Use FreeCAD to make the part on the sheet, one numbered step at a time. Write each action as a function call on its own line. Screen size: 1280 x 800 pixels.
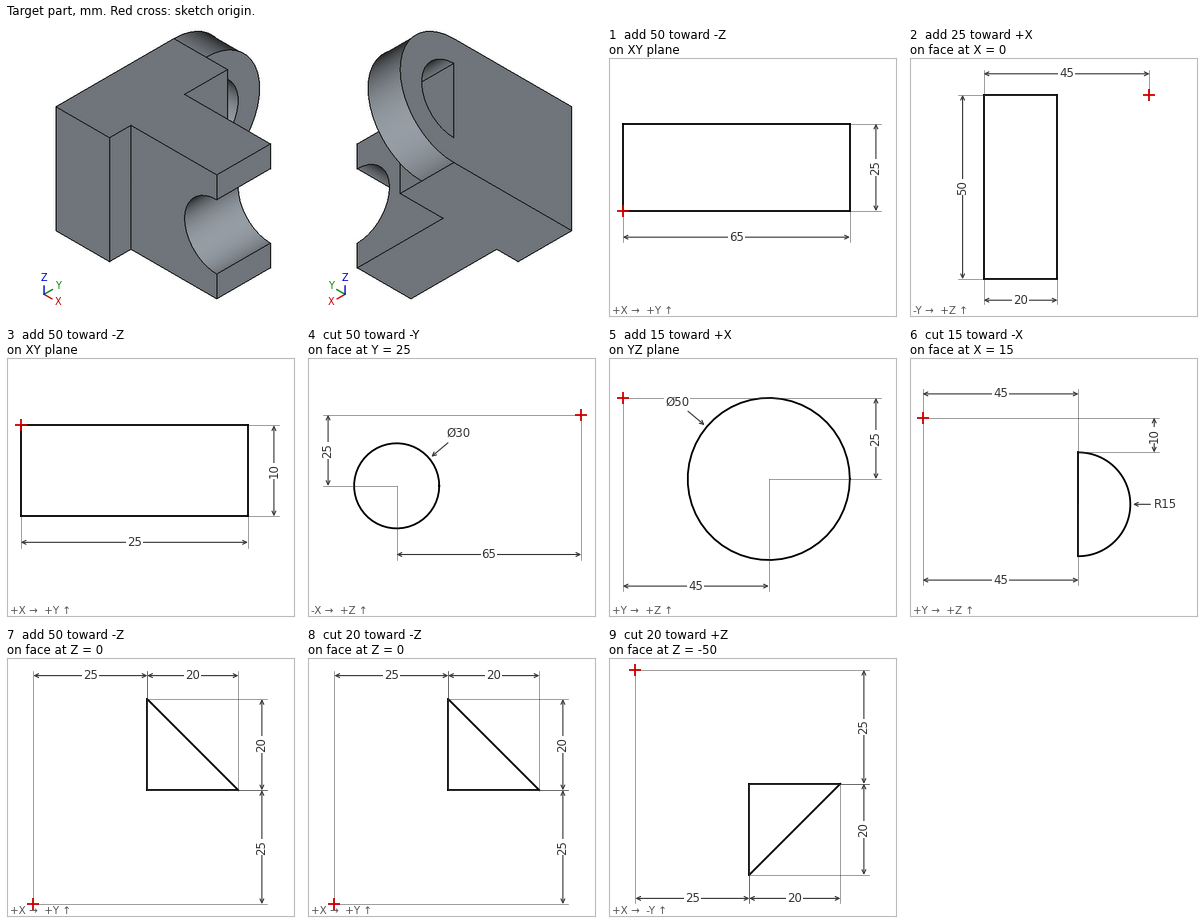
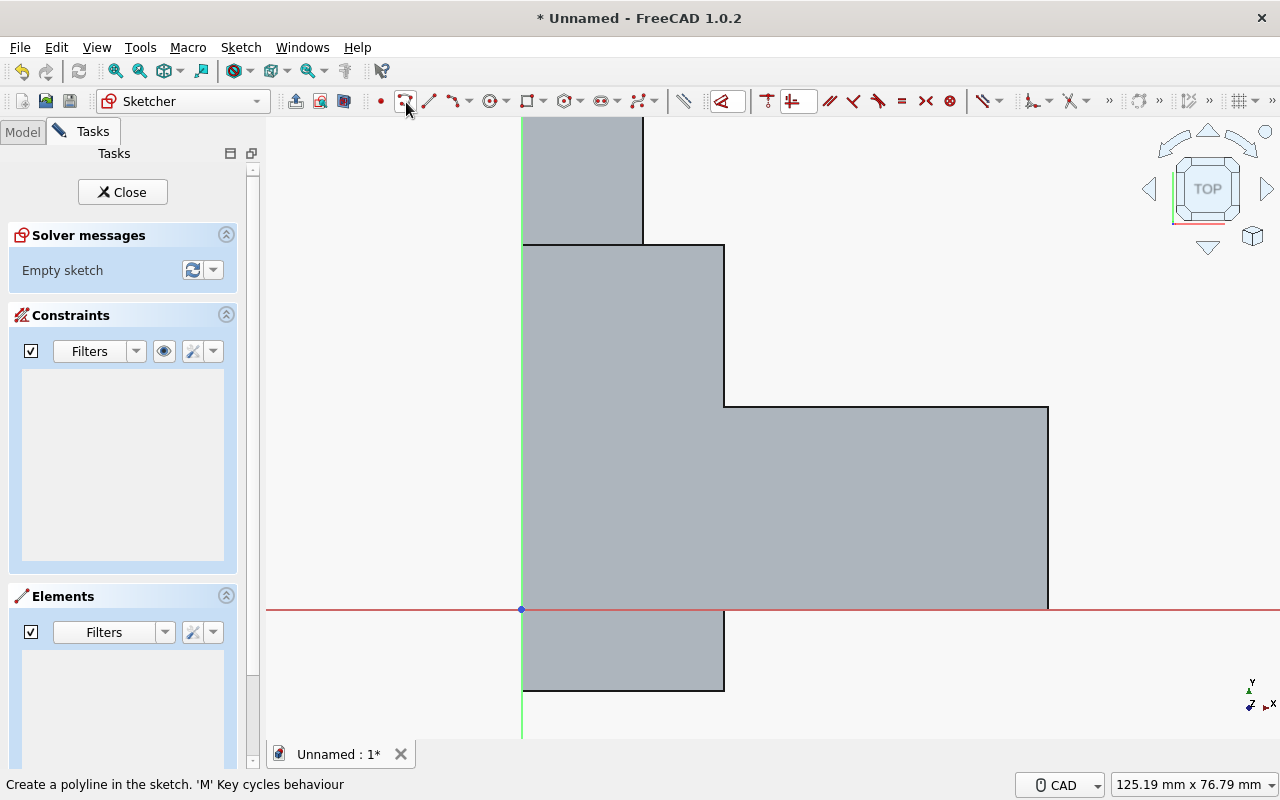
click(724, 407)
click(886, 407)
click(724, 245)
click(724, 408)
key(Escape)
key(Escape)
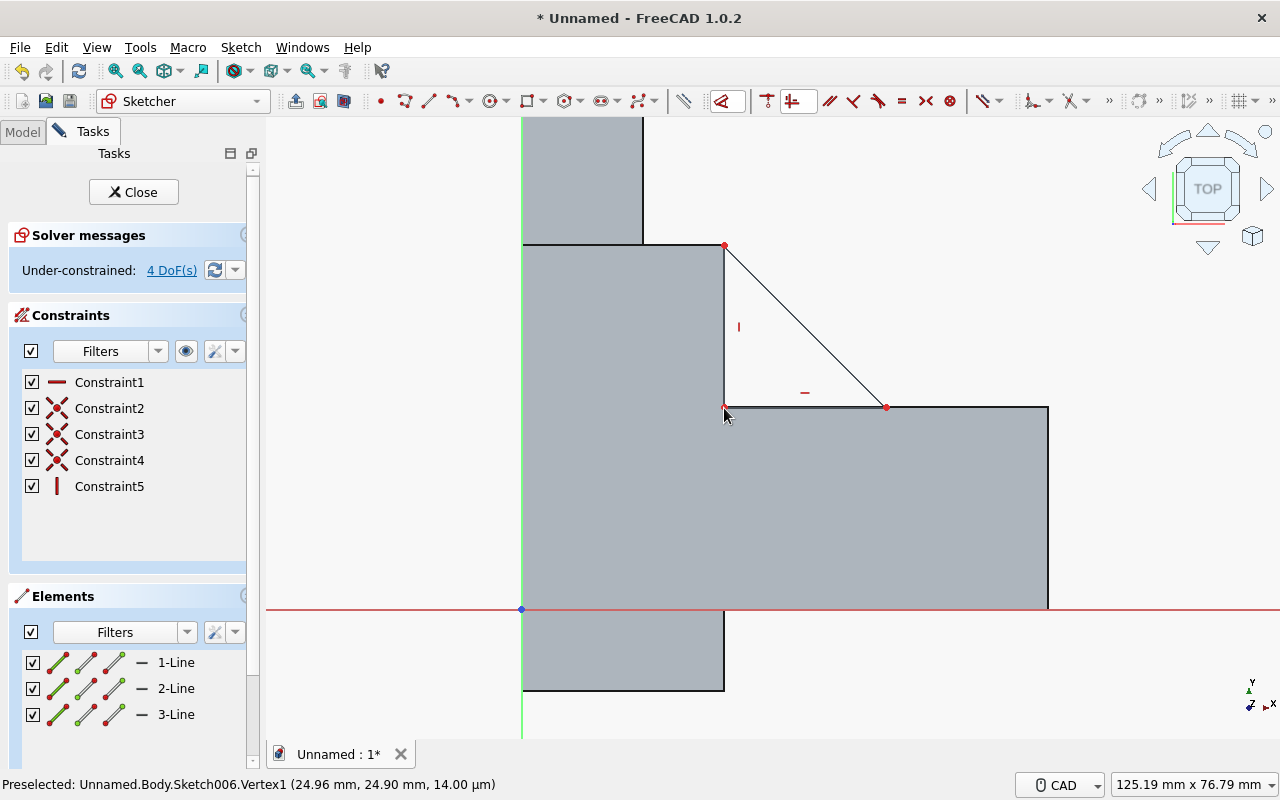
click(773, 408)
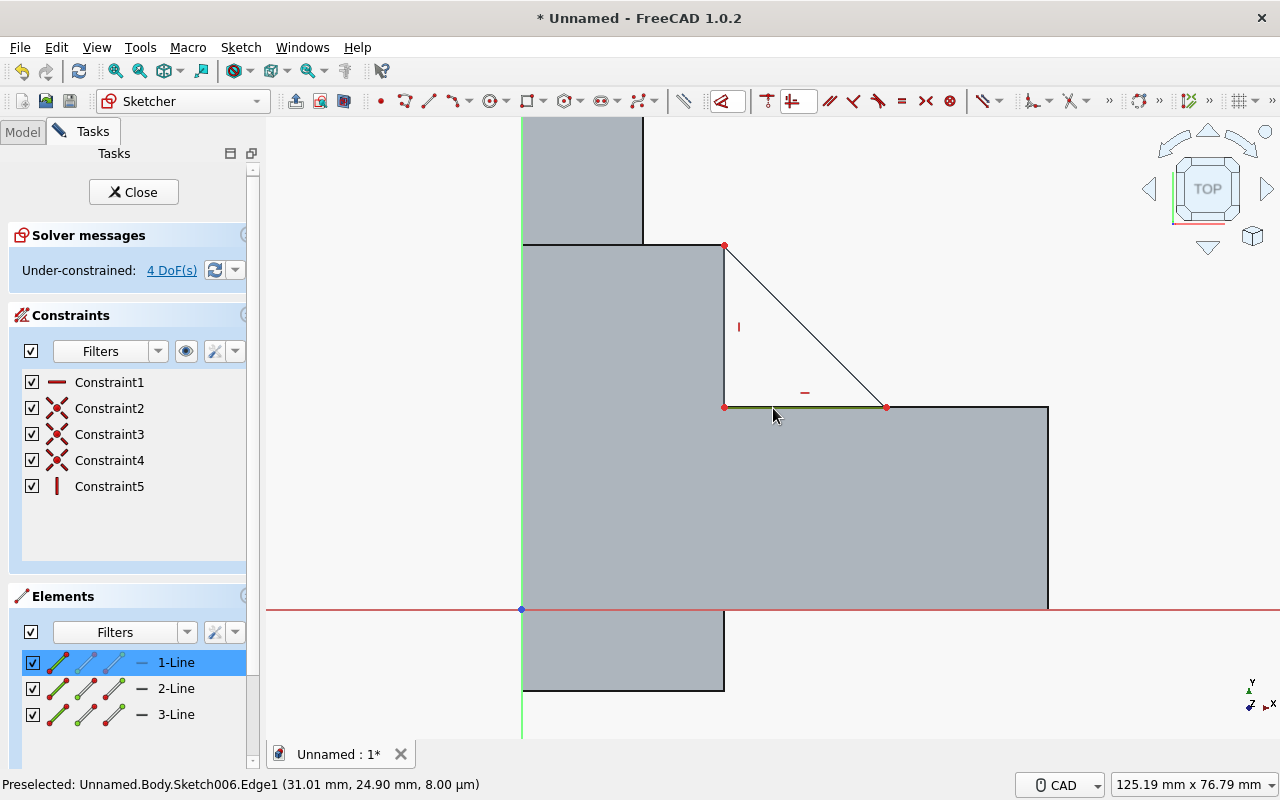
key(l)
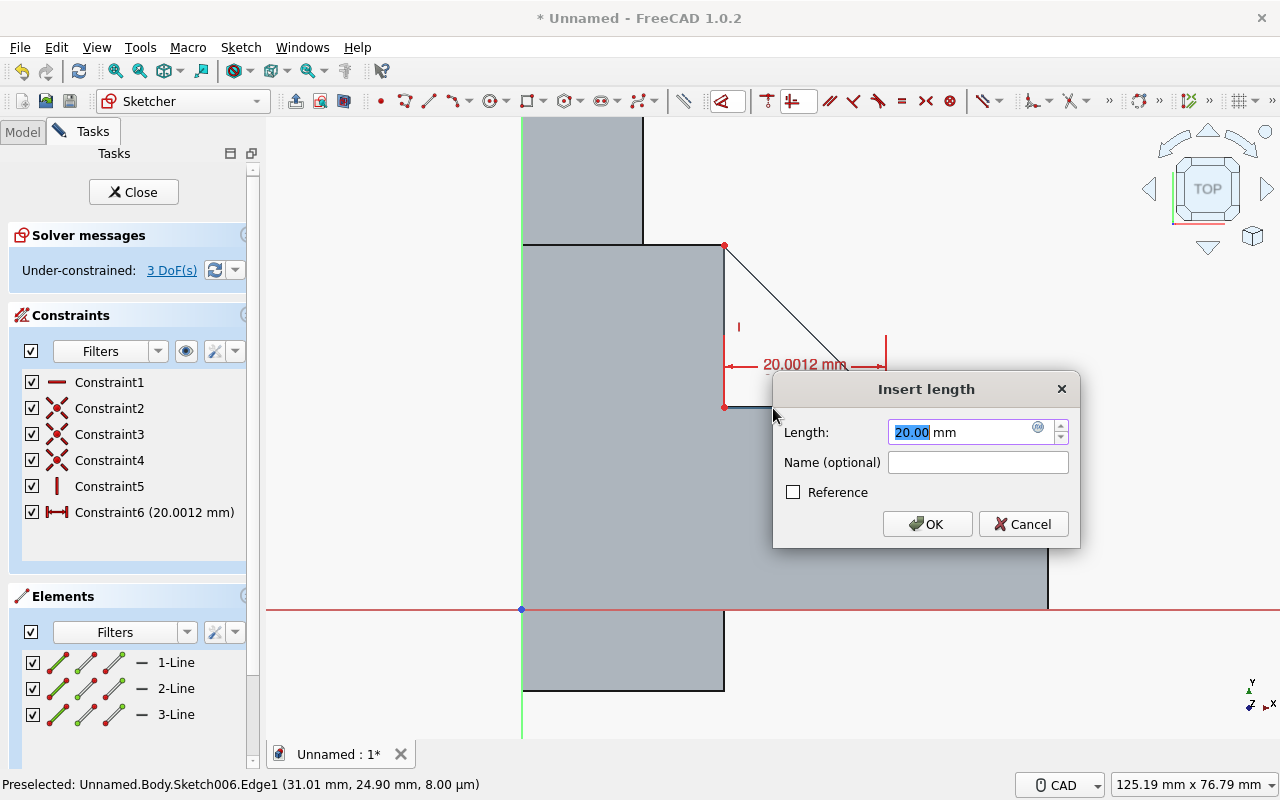
text(20)
key(Return)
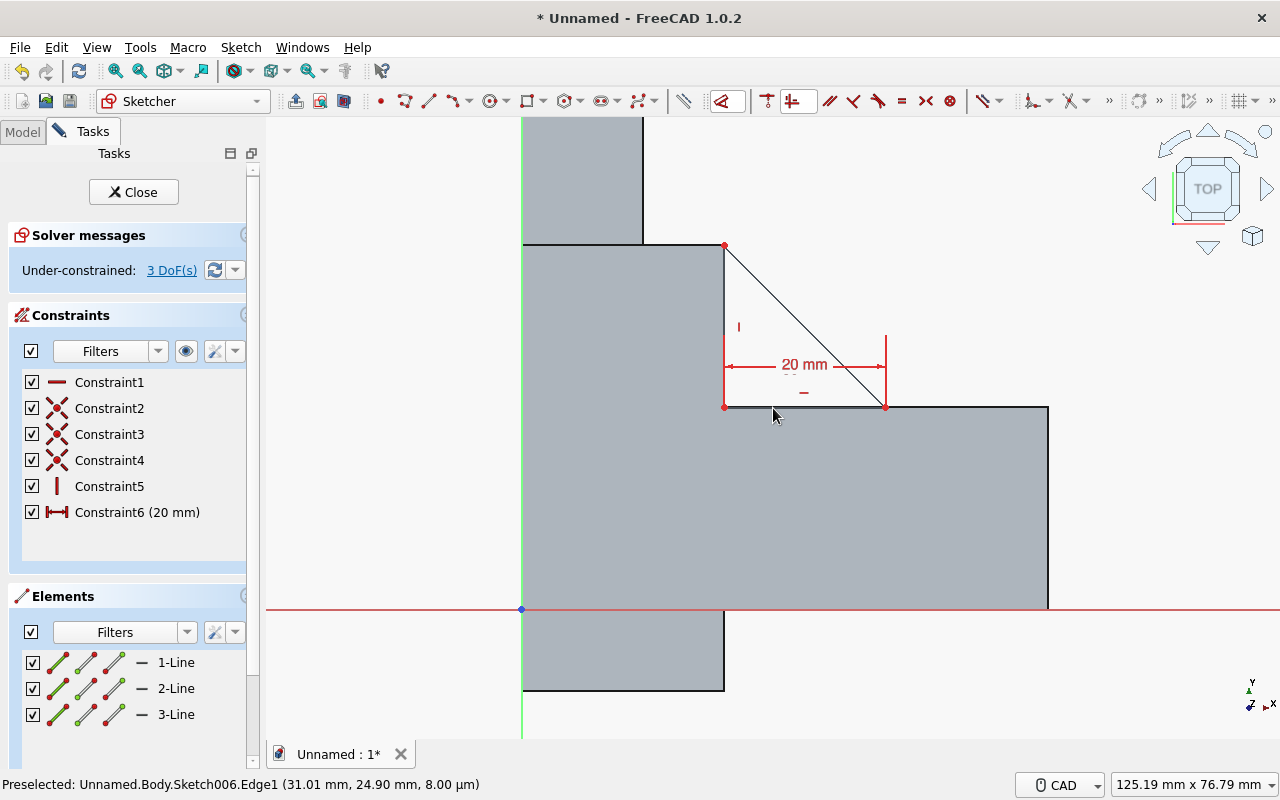
click(724, 295)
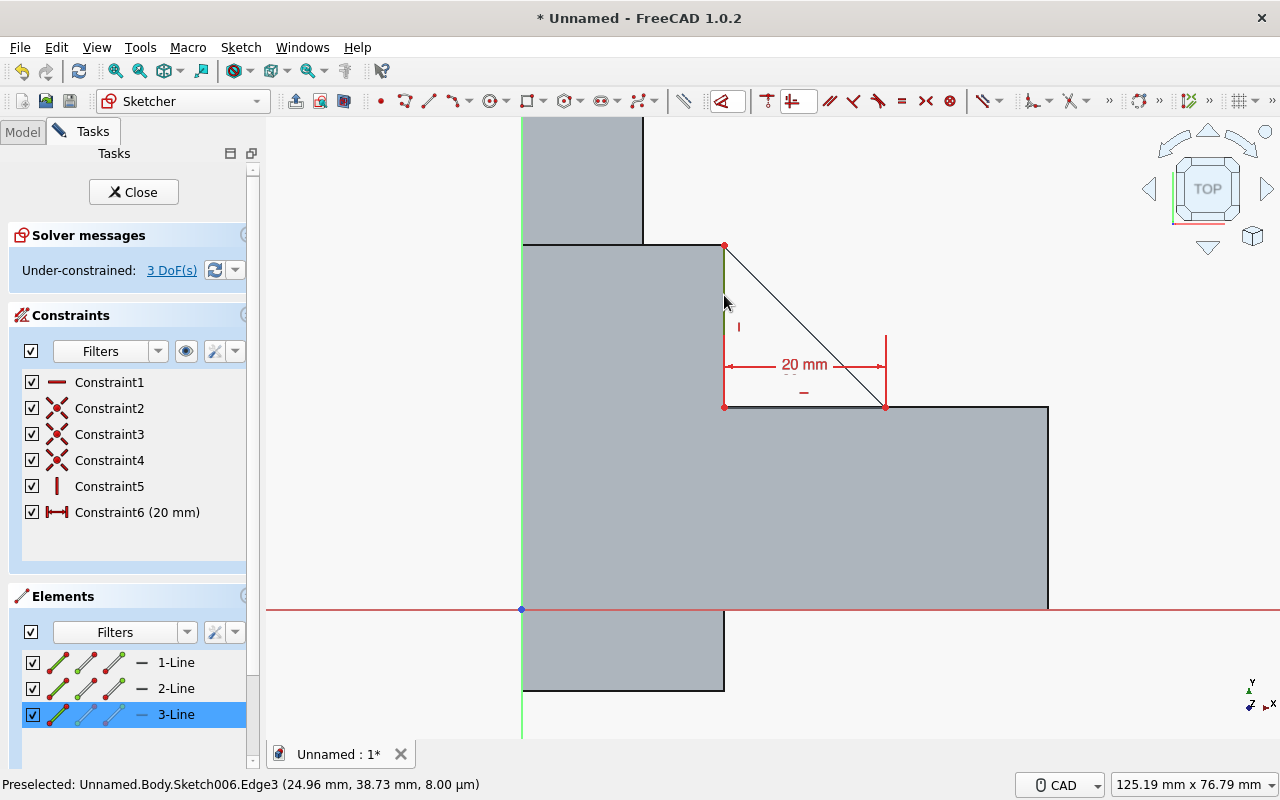
key(i)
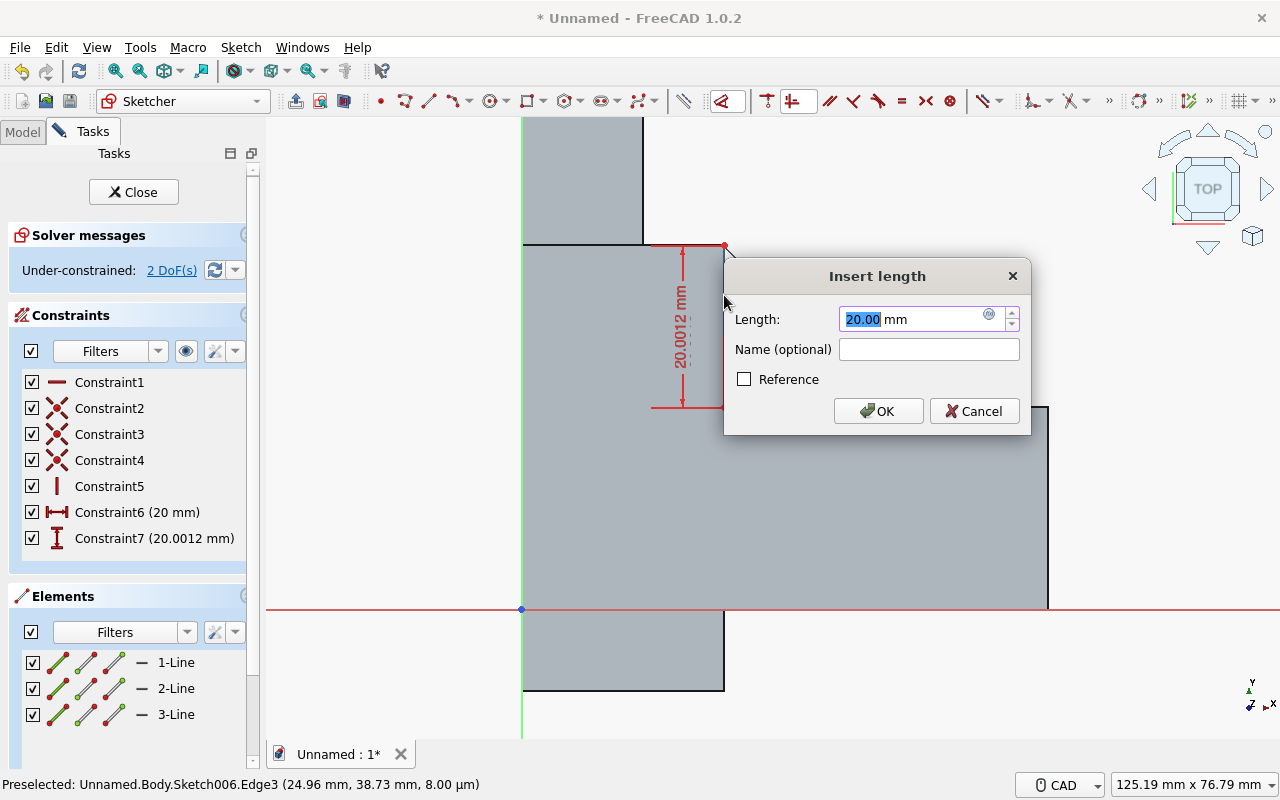
text(20)
key(Return)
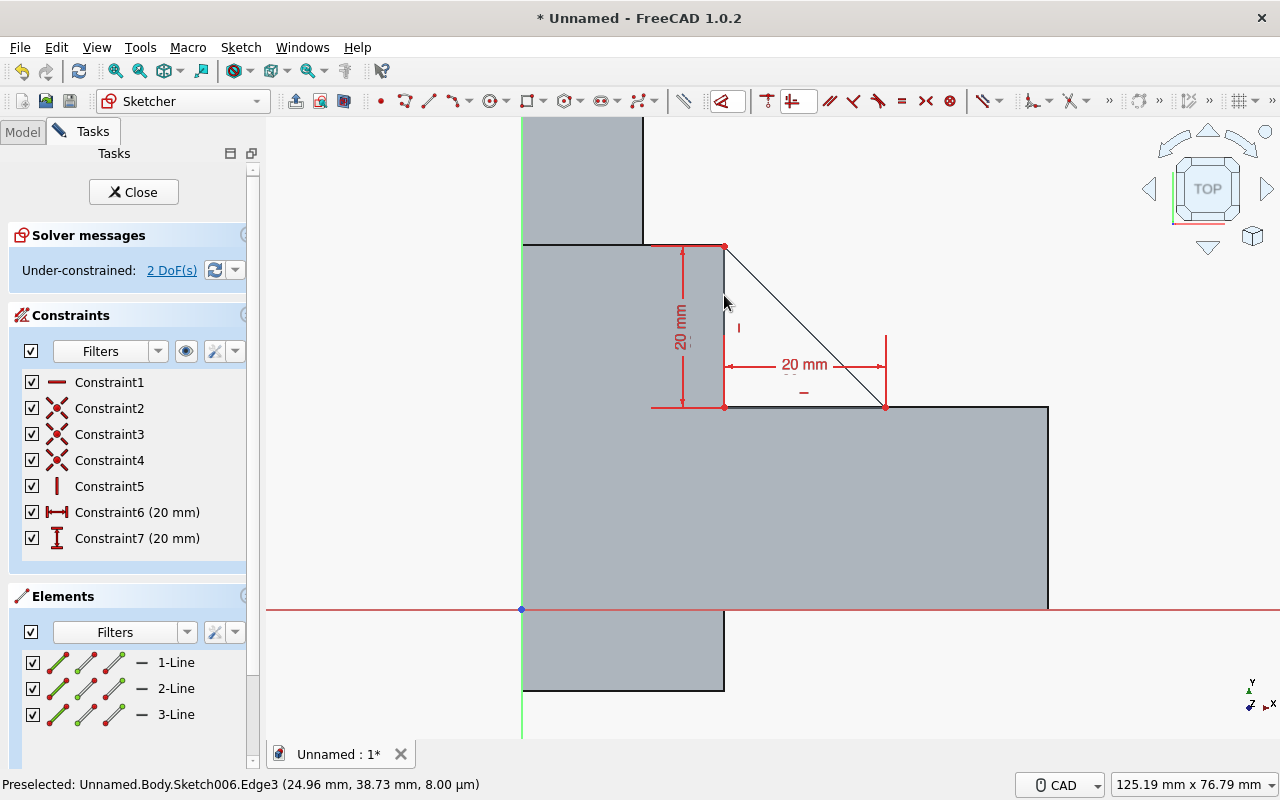
click(724, 408)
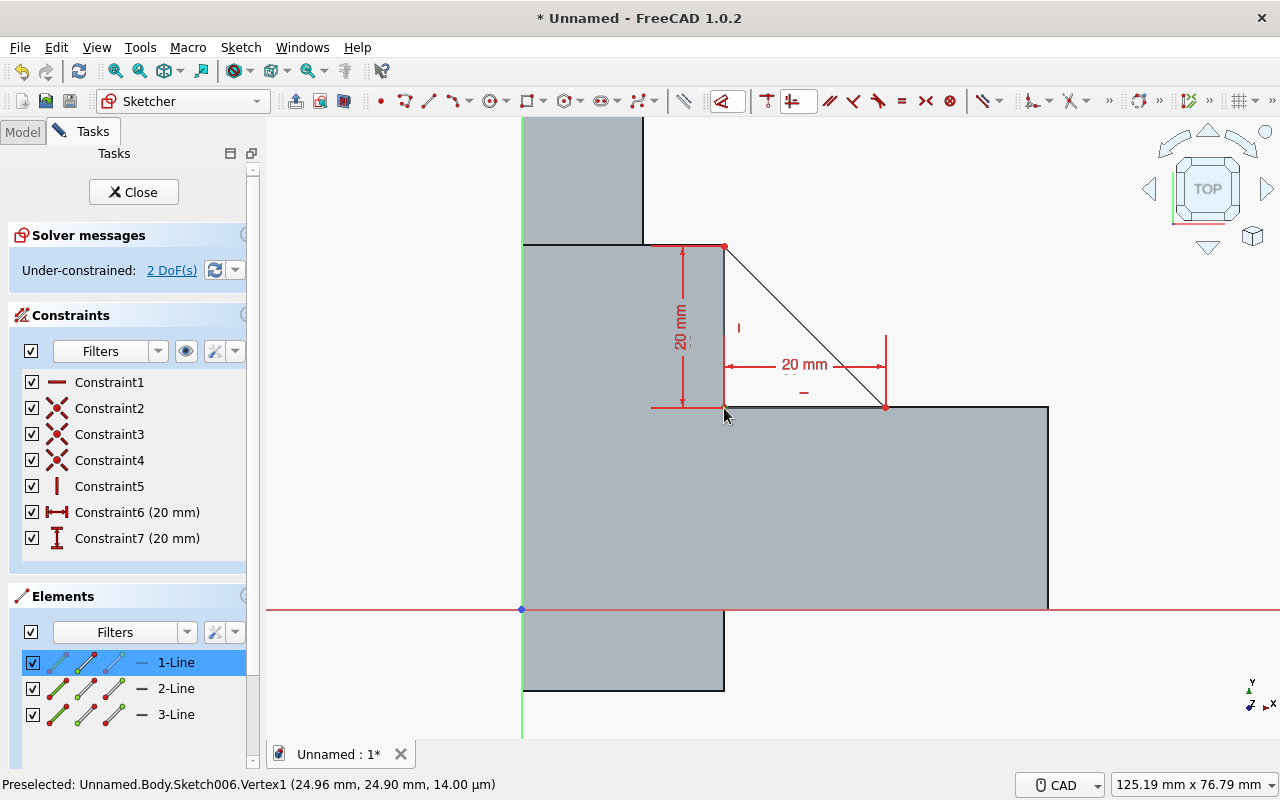
click(740, 102)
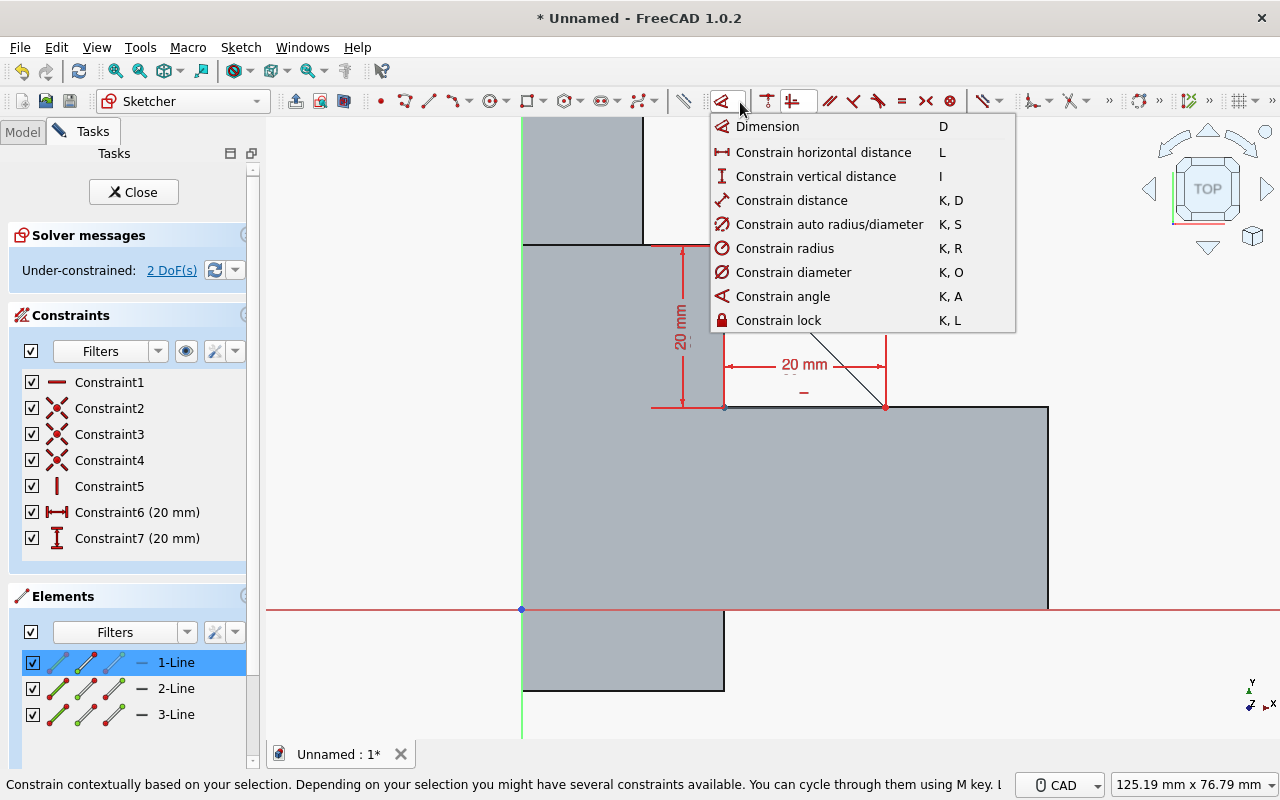
click(863, 152)